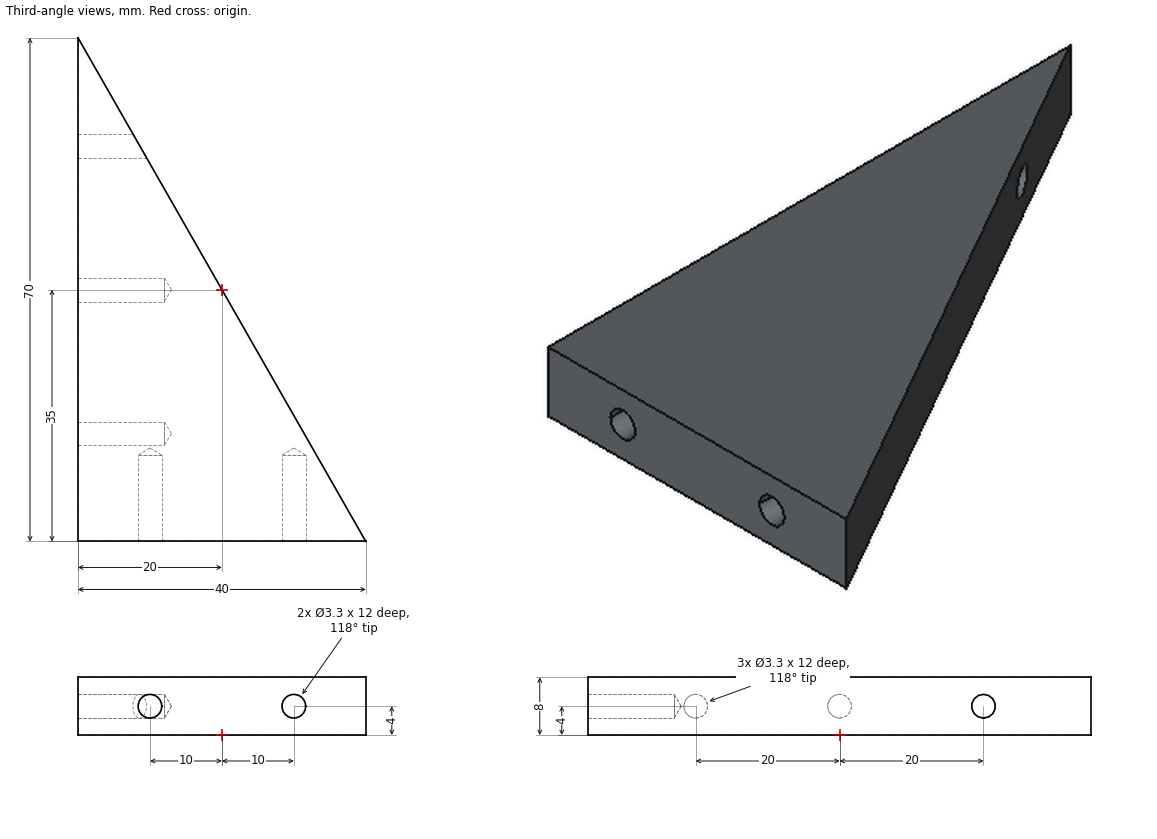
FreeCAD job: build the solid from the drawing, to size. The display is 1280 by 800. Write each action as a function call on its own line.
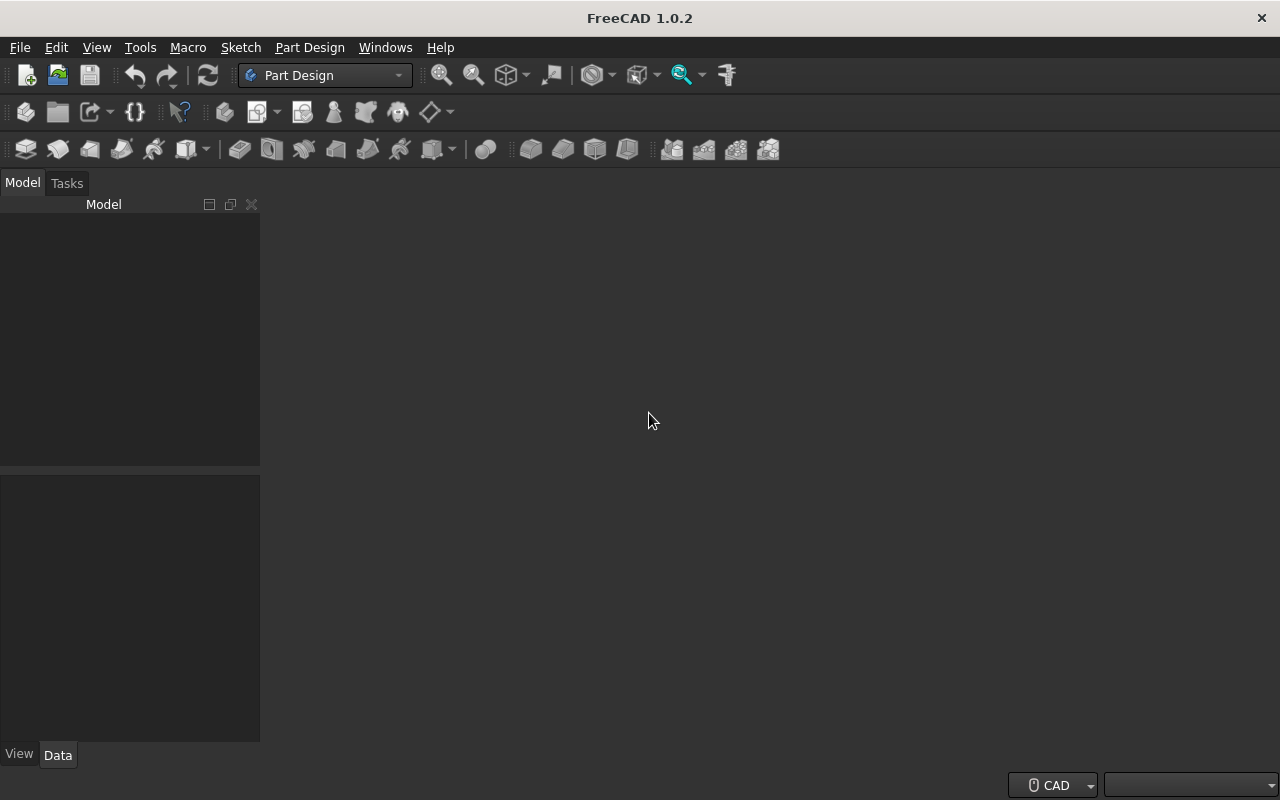
click(26, 76)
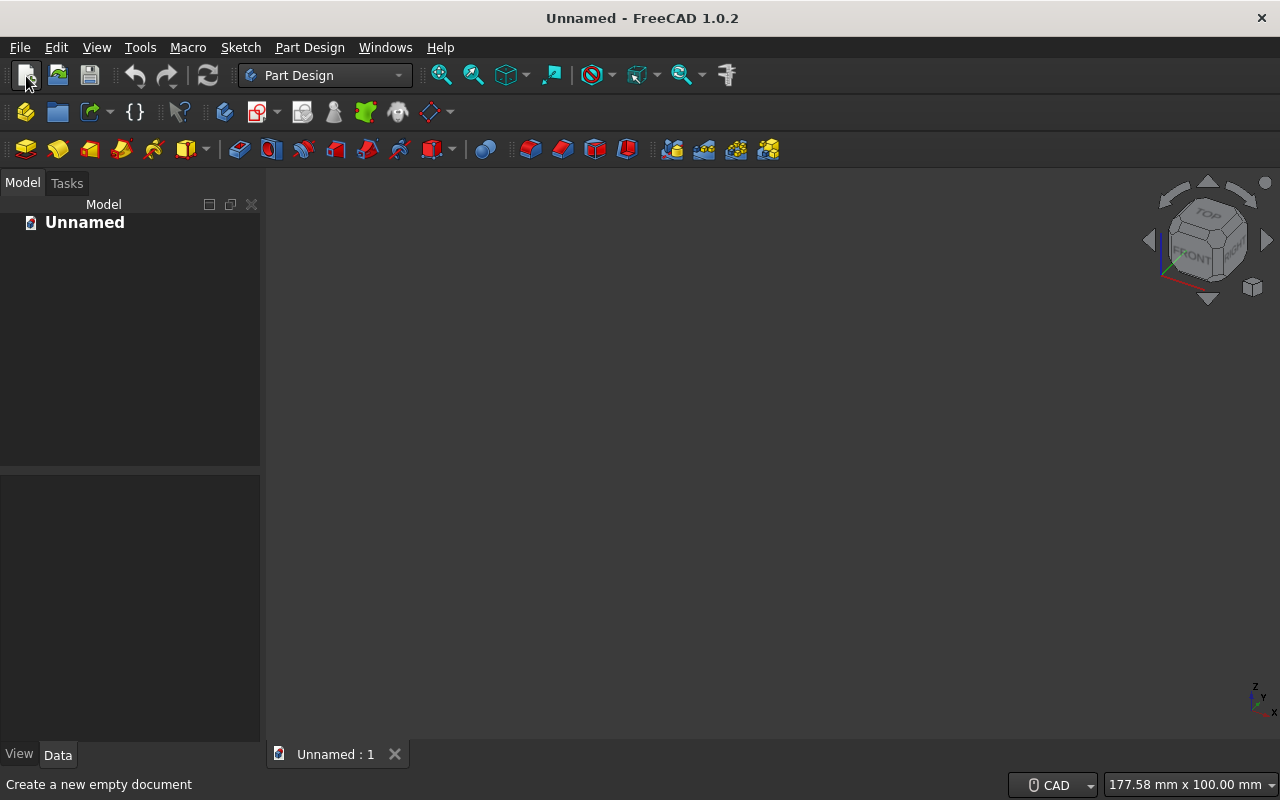
click(258, 112)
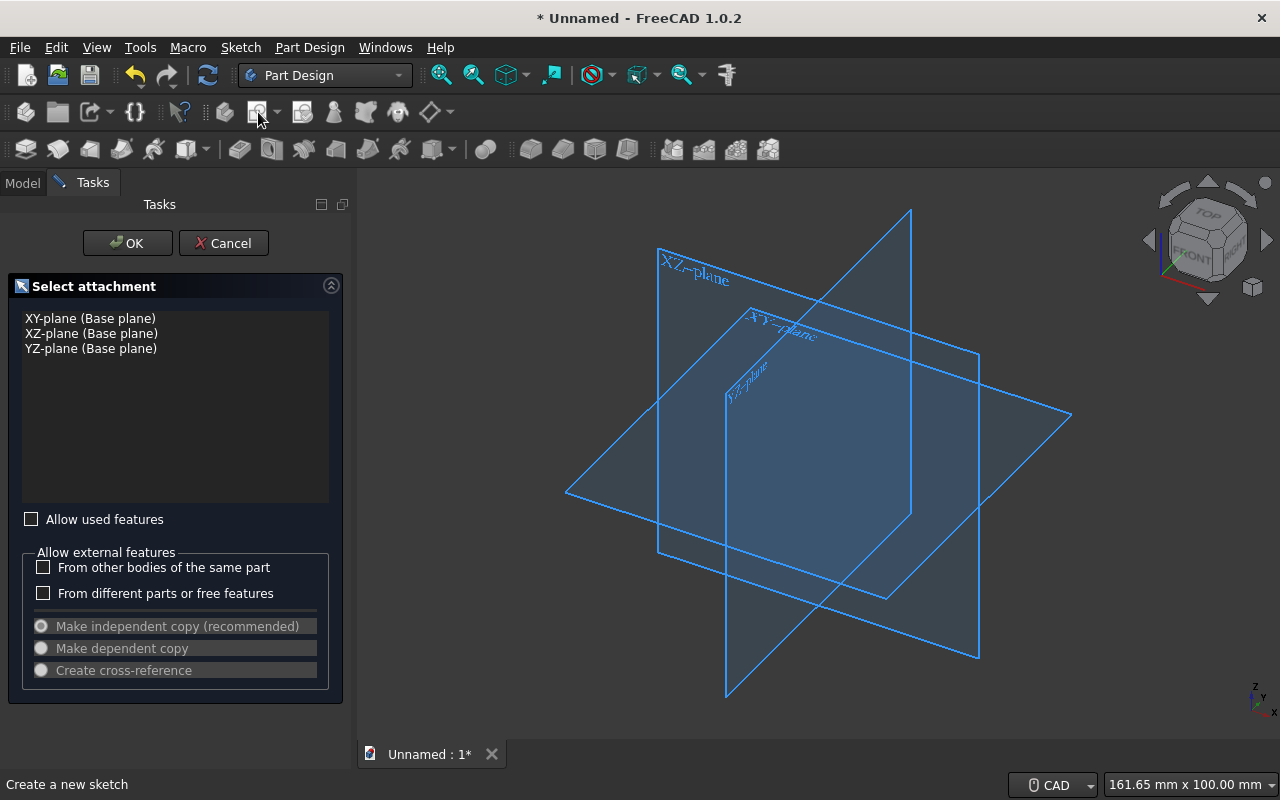
click(82, 318)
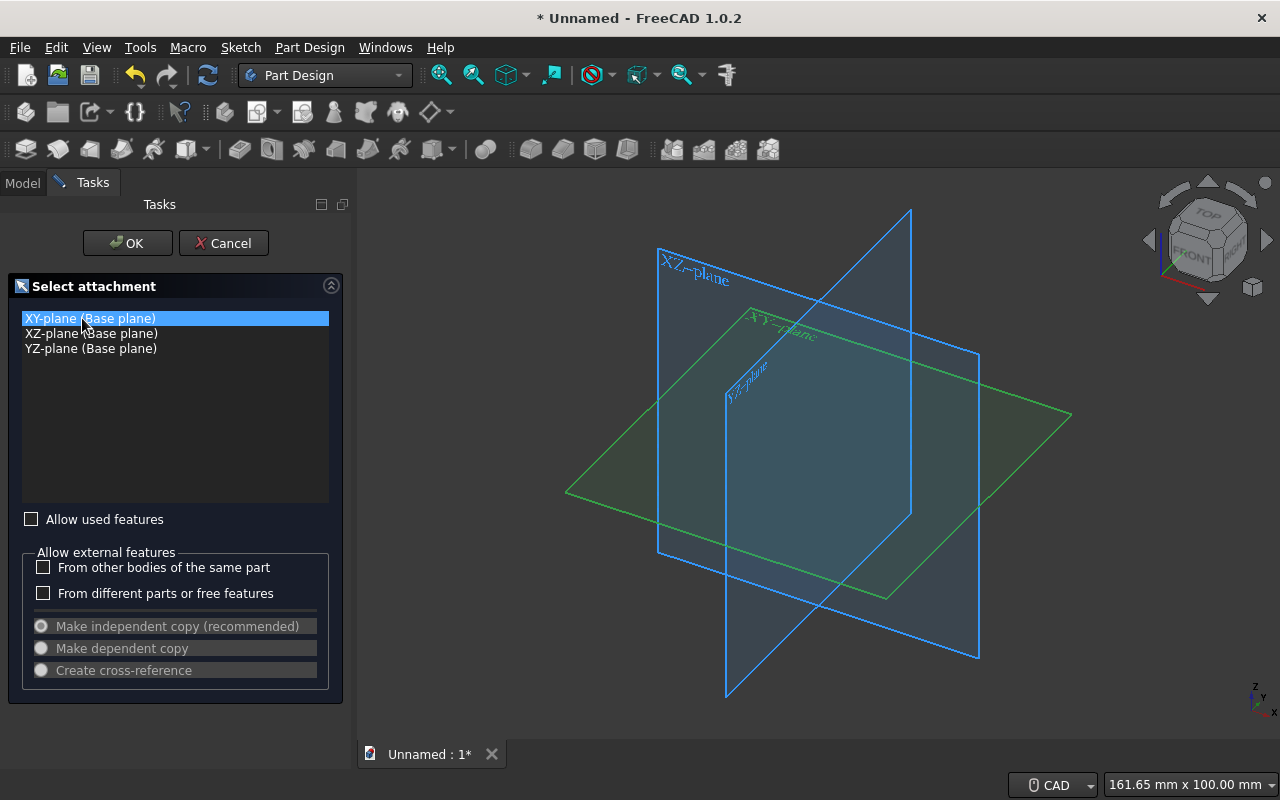
click(128, 243)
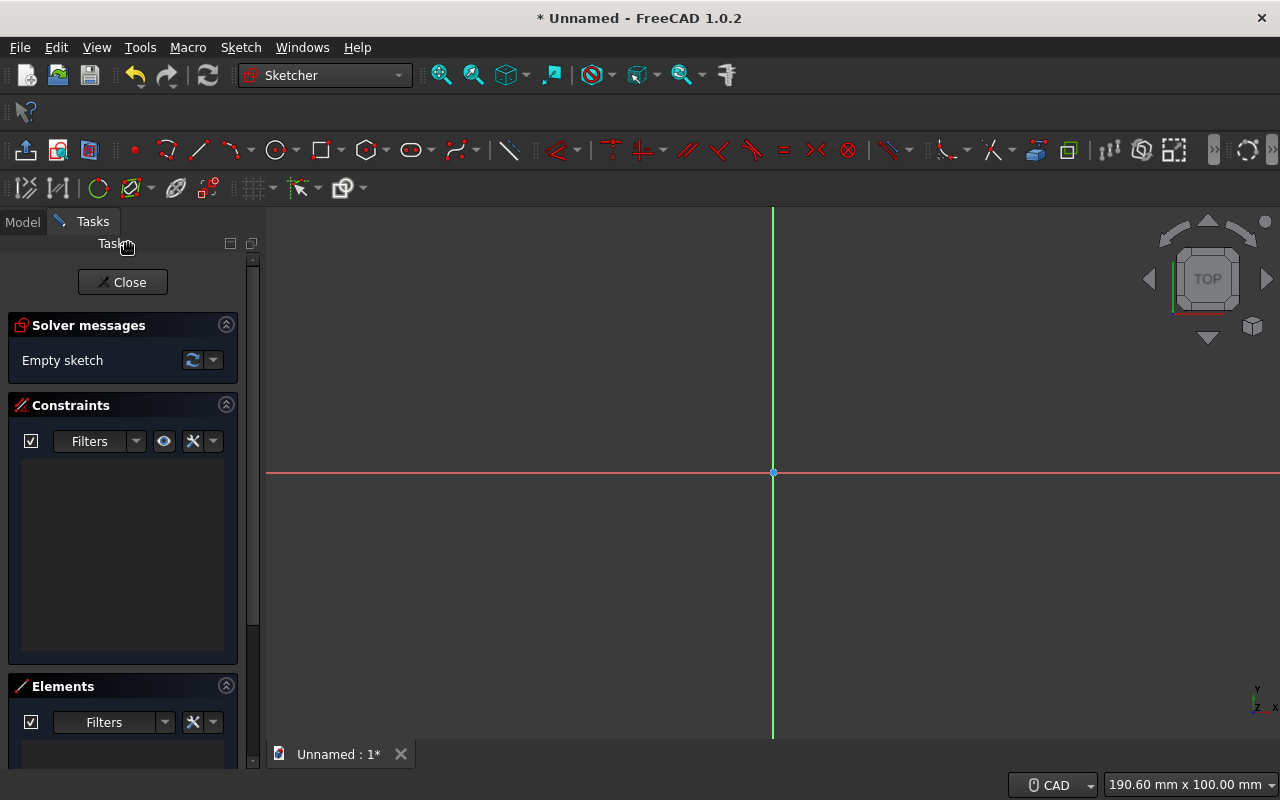
click(168, 150)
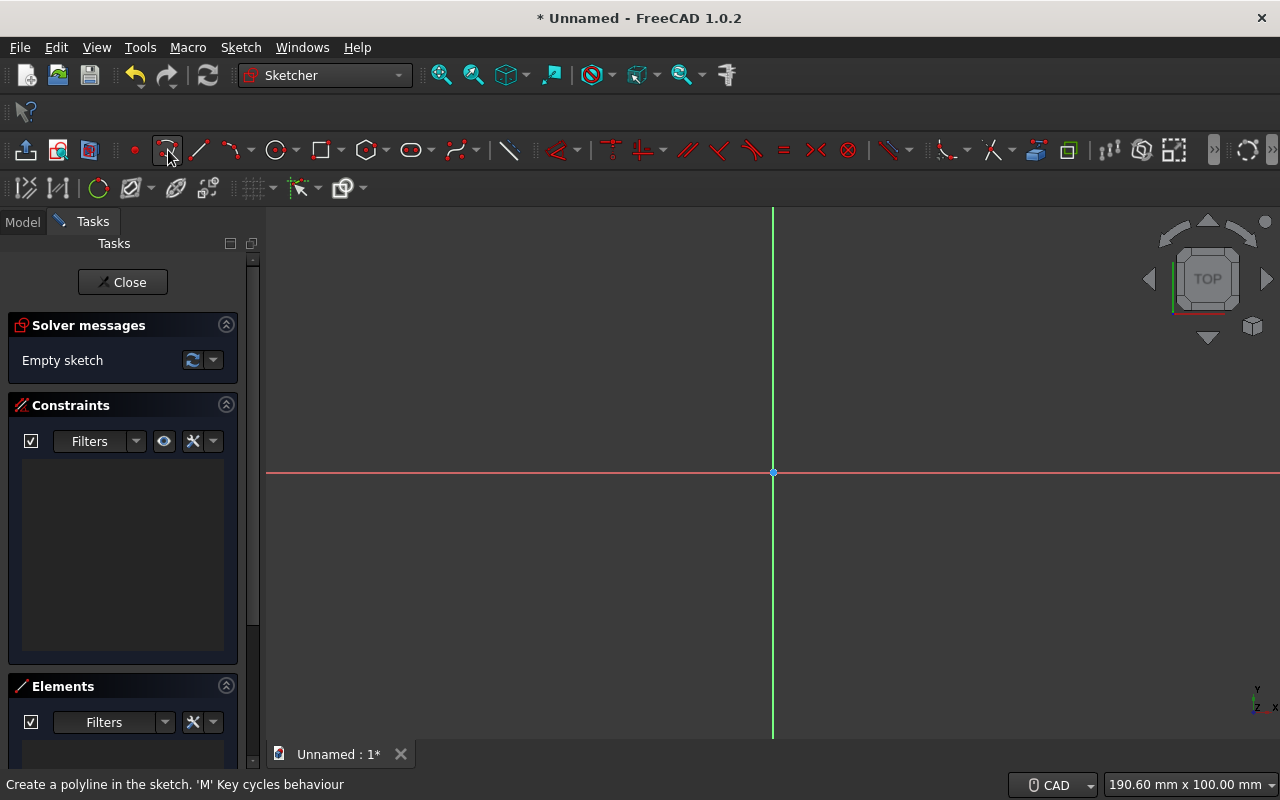
click(667, 659)
click(879, 659)
click(667, 287)
click(667, 660)
key(Escape)
key(Escape)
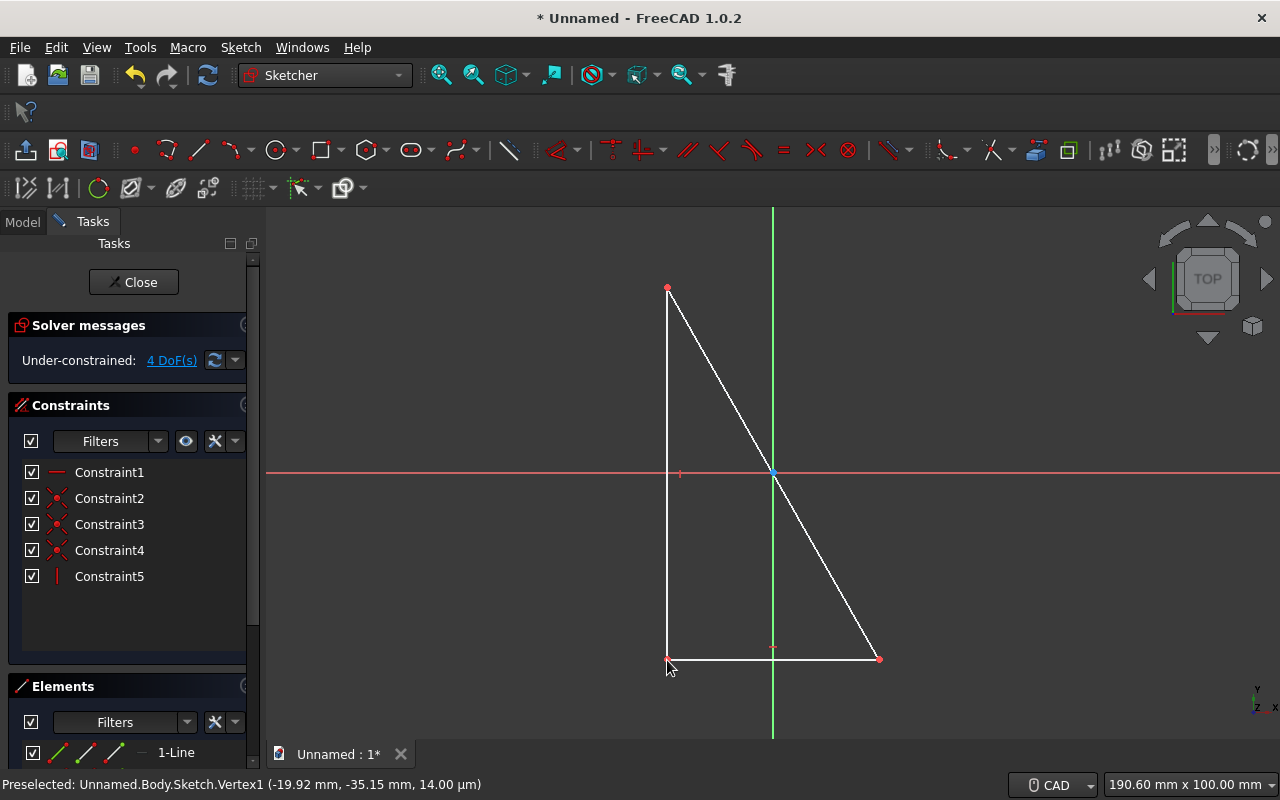
click(731, 660)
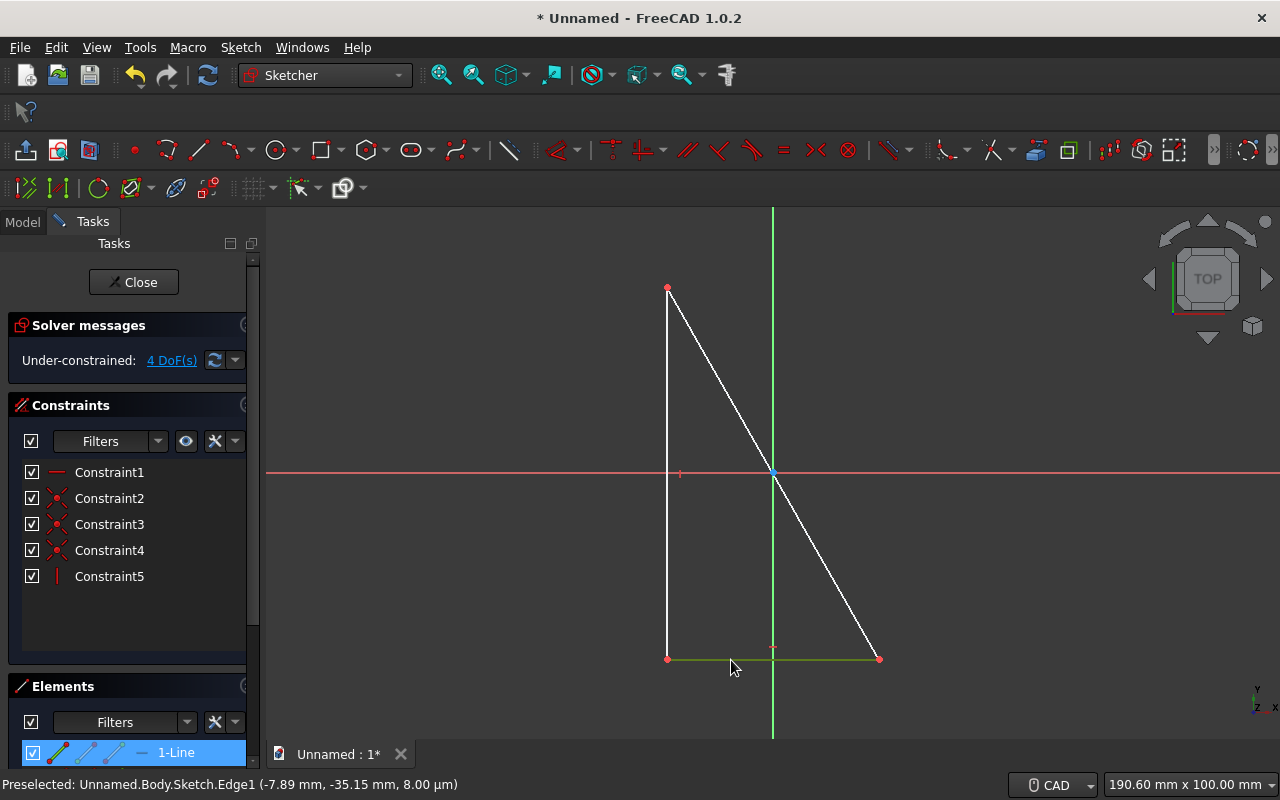
click(580, 150)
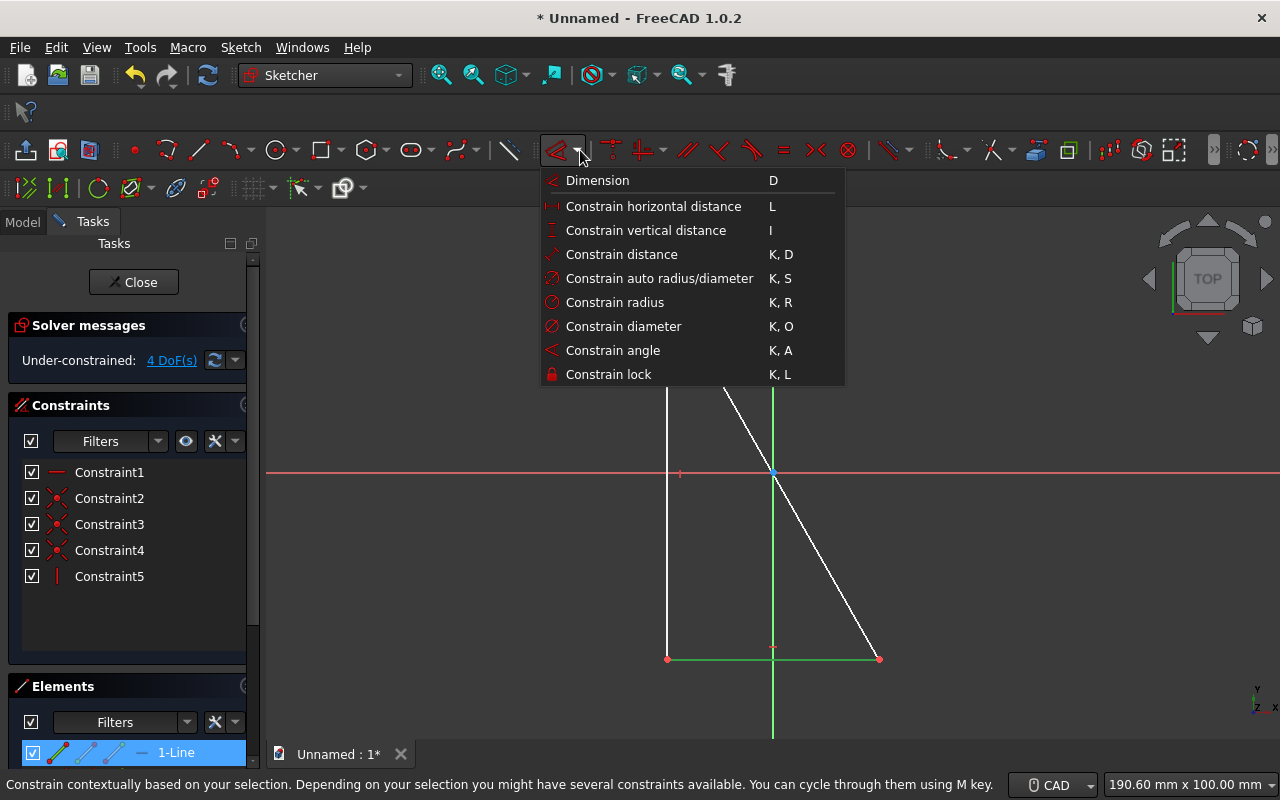
click(693, 206)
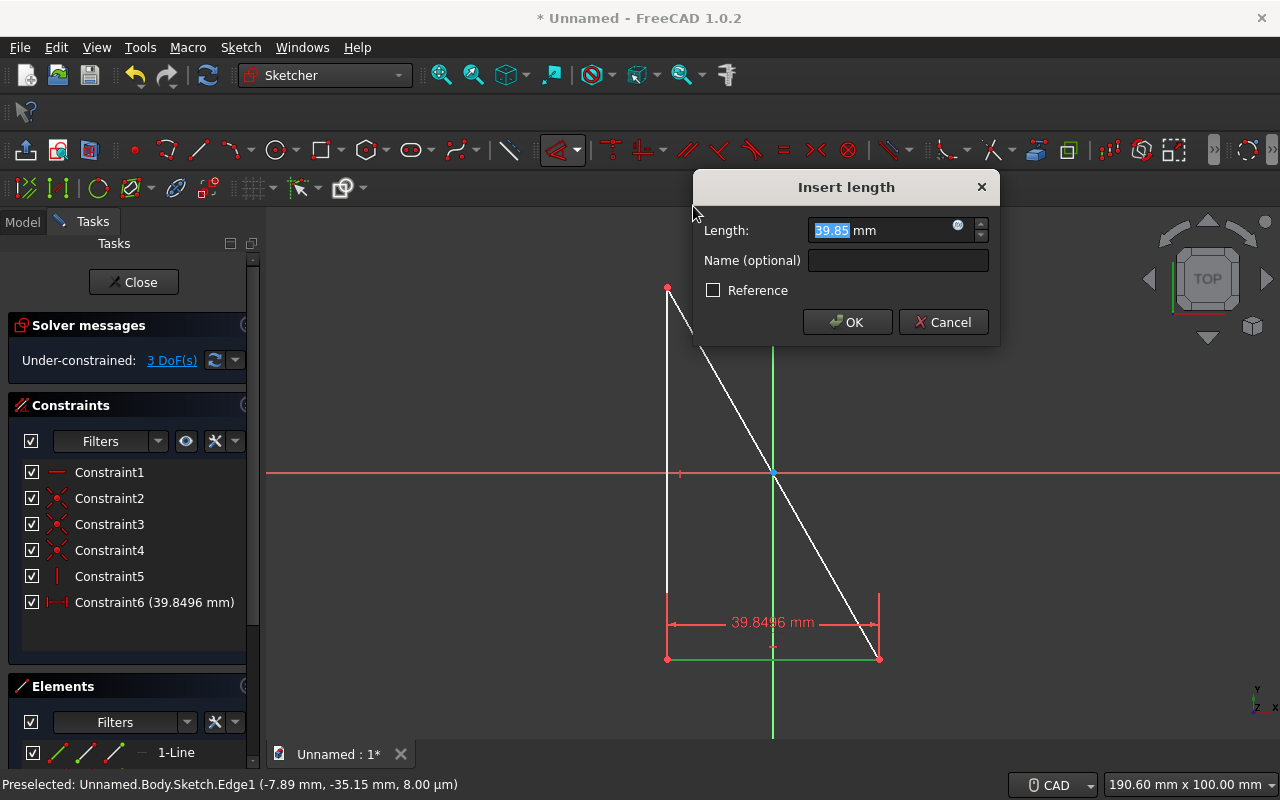
text(40)
key(Return)